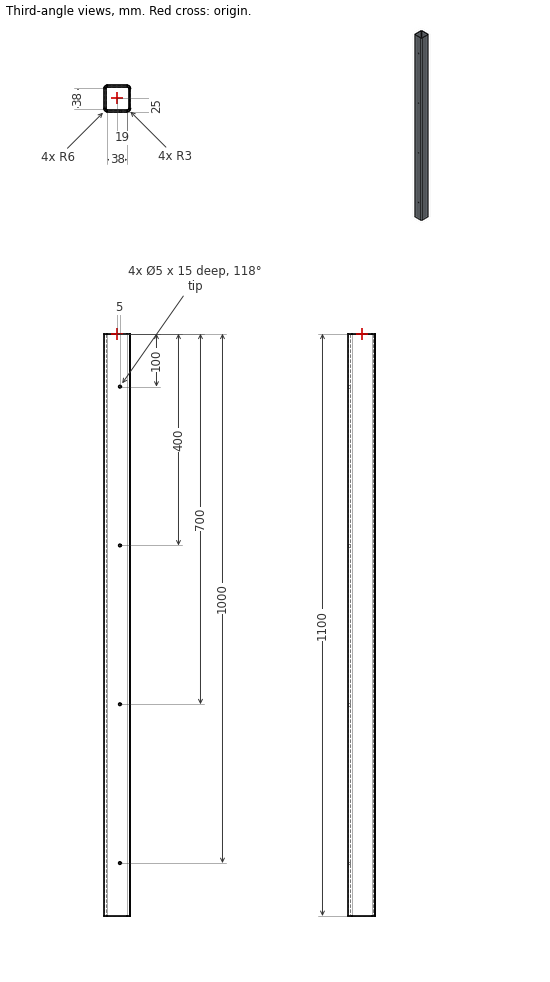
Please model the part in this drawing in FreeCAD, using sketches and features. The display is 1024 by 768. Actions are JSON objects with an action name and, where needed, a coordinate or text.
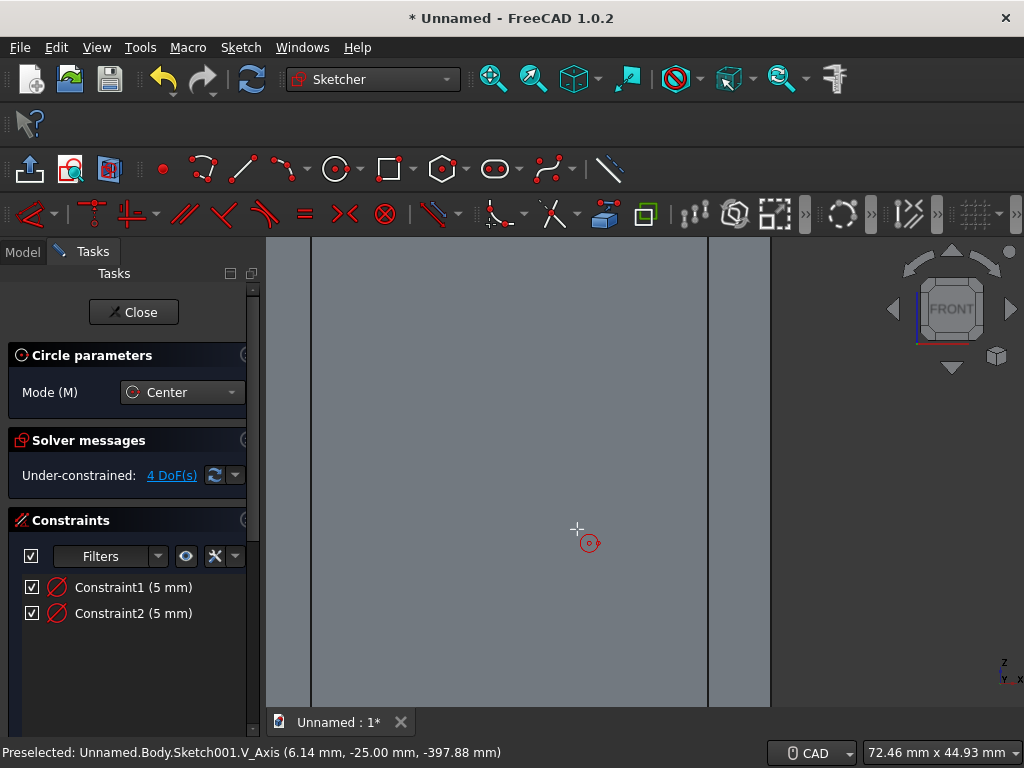
{"action": "scroll", "coordinate": [577, 542], "scroll_direction": "down", "scroll_amount": 17}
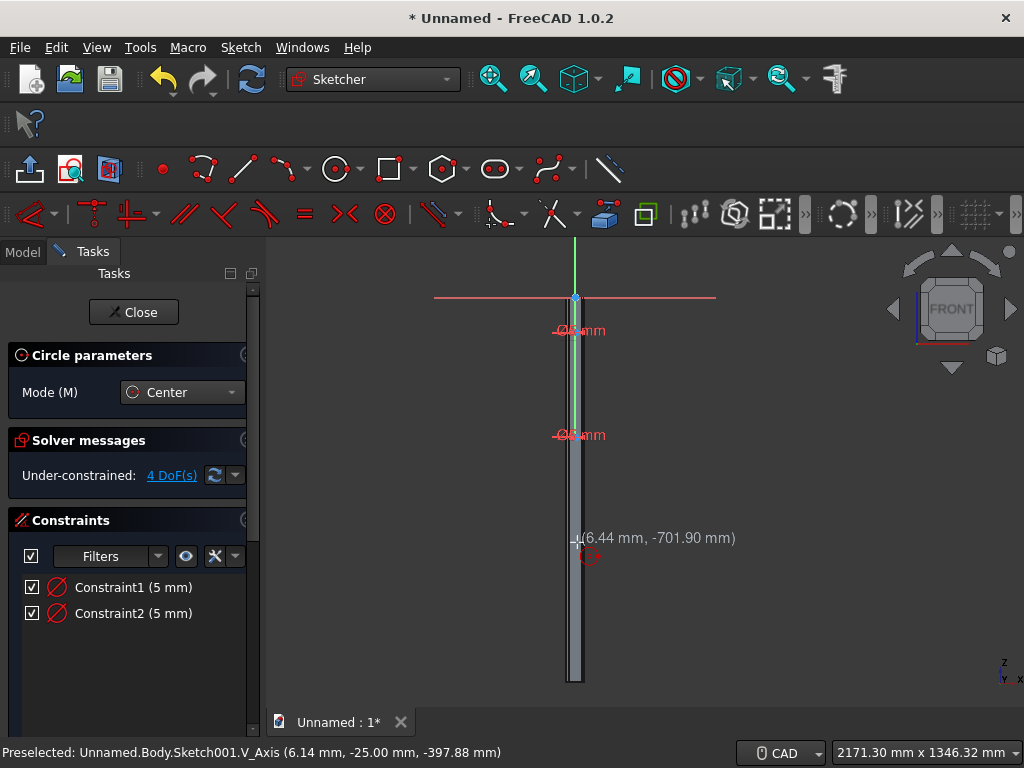
{"action": "scroll", "coordinate": [577, 542], "scroll_direction": "up", "scroll_amount": 12}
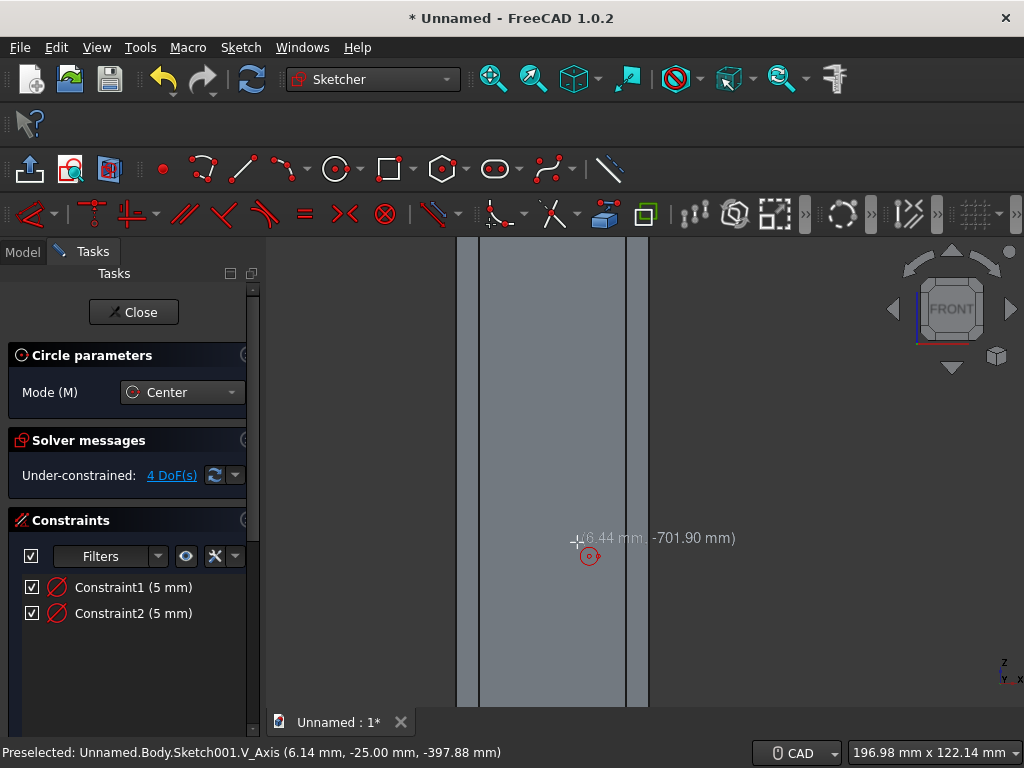
{"action": "left_click", "coordinate": [572, 535]}
{"action": "mouse_move", "coordinate": [579, 529]}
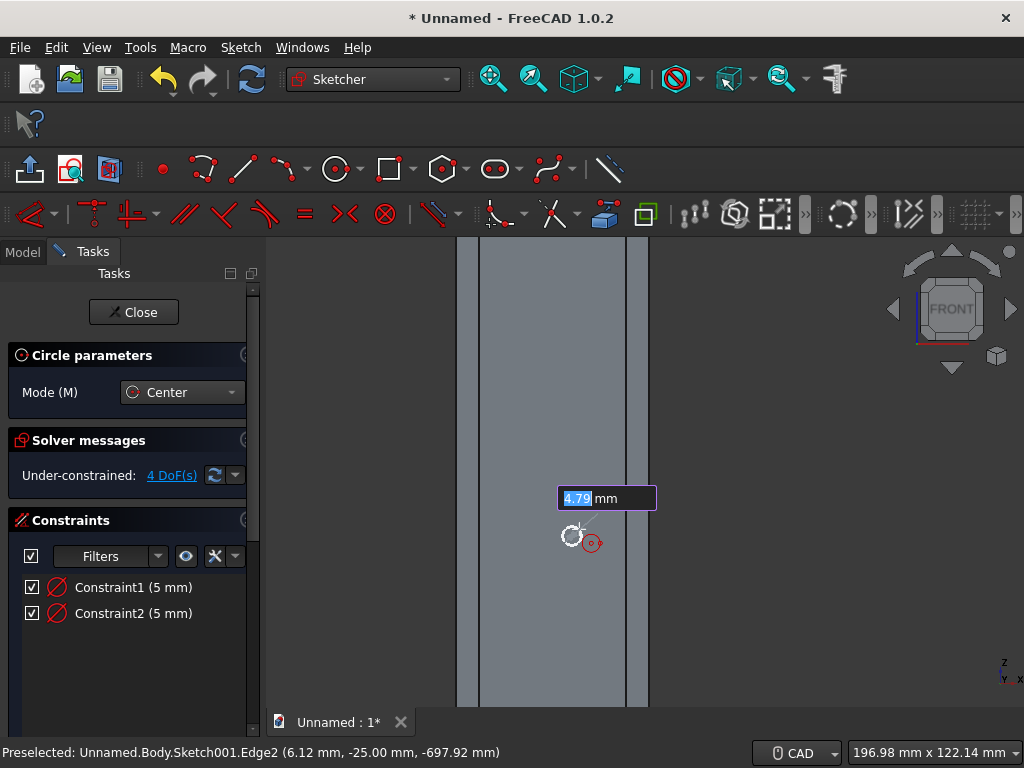
{"action": "type", "text": "5"}
{"action": "key", "text": "Return"}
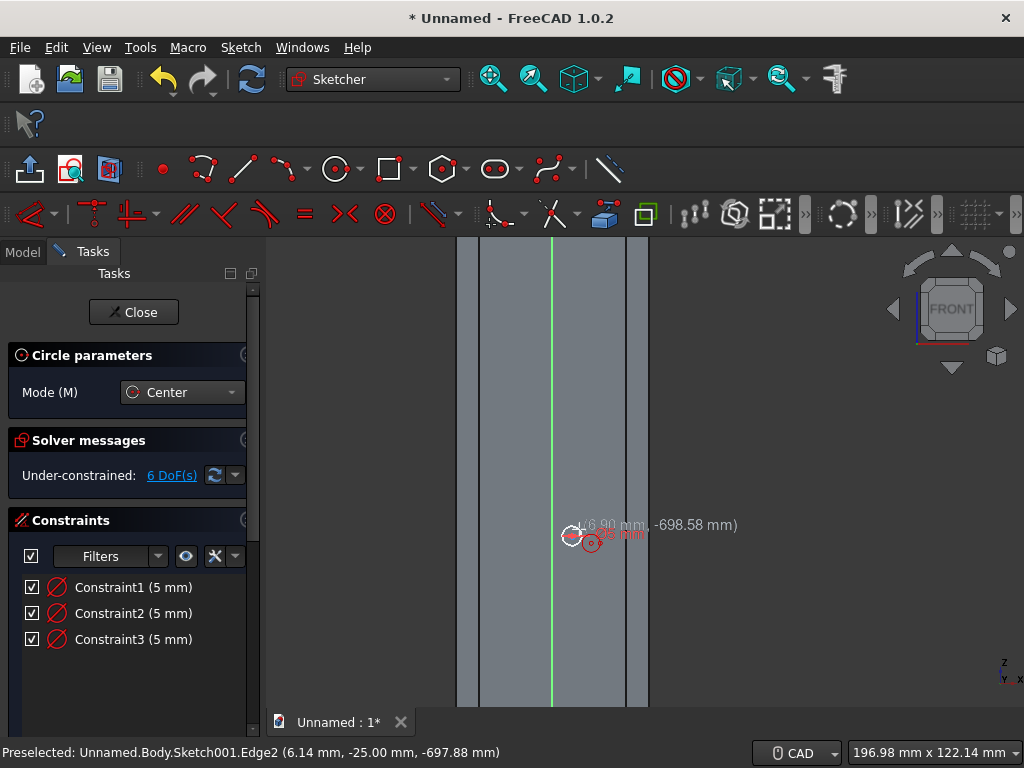
{"action": "scroll", "coordinate": [577, 528], "scroll_direction": "down", "scroll_amount": 13}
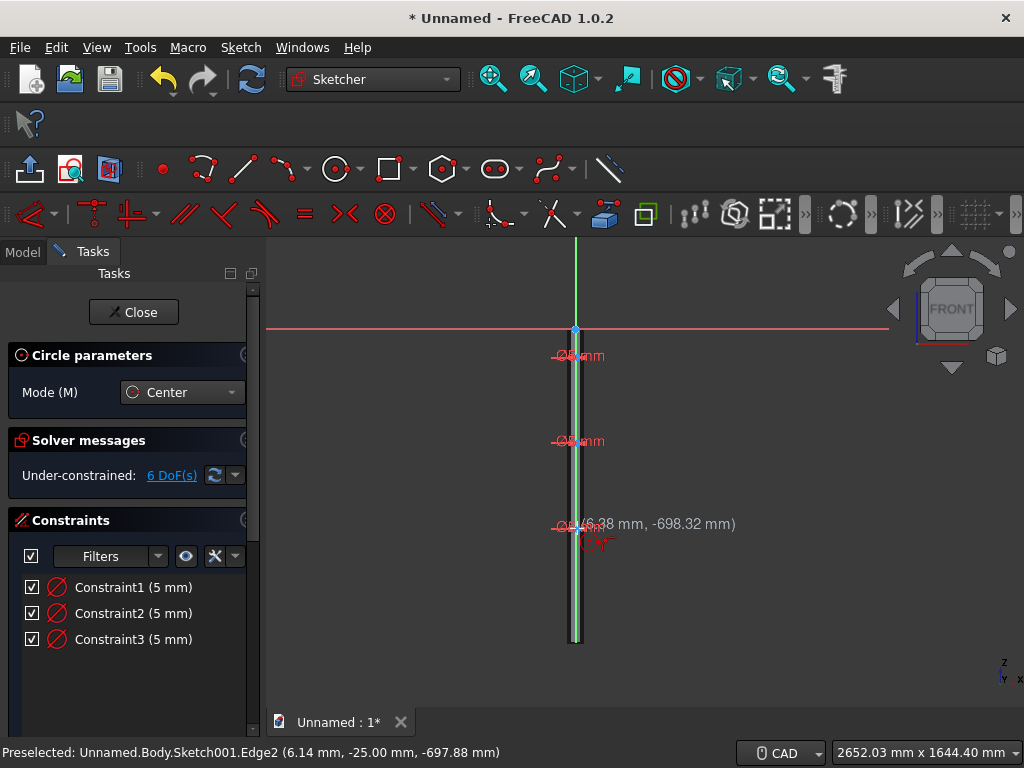
{"action": "scroll", "coordinate": [577, 615], "scroll_direction": "up", "scroll_amount": 18}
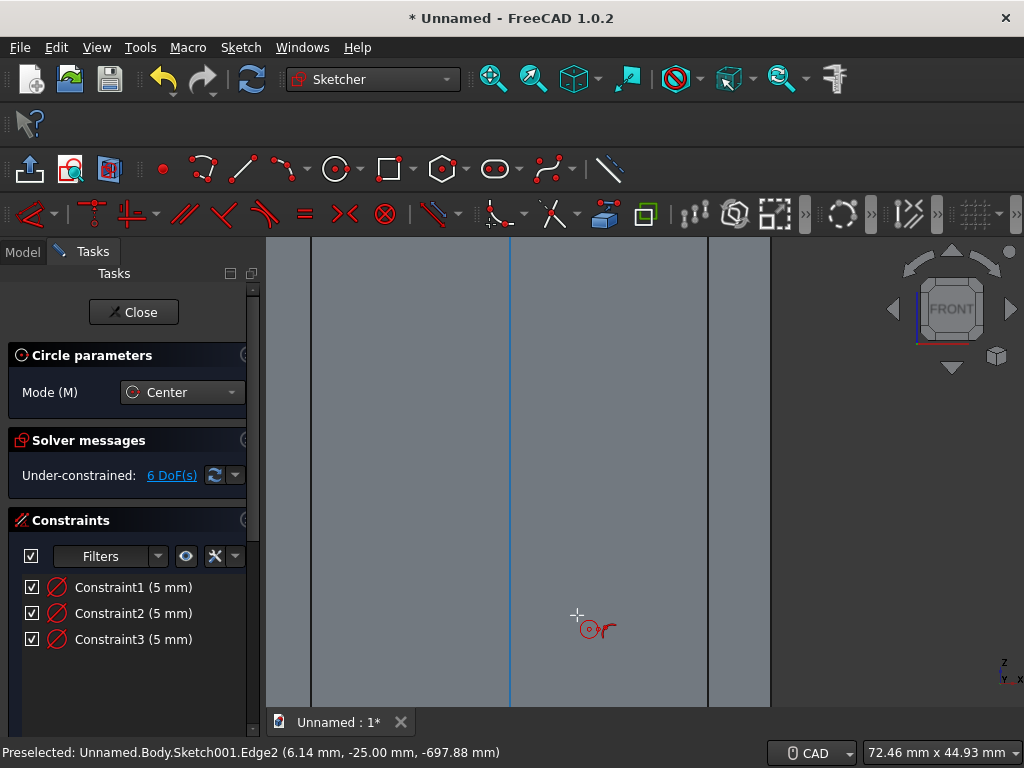
{"action": "scroll", "coordinate": [577, 648], "scroll_direction": "down", "scroll_amount": 17}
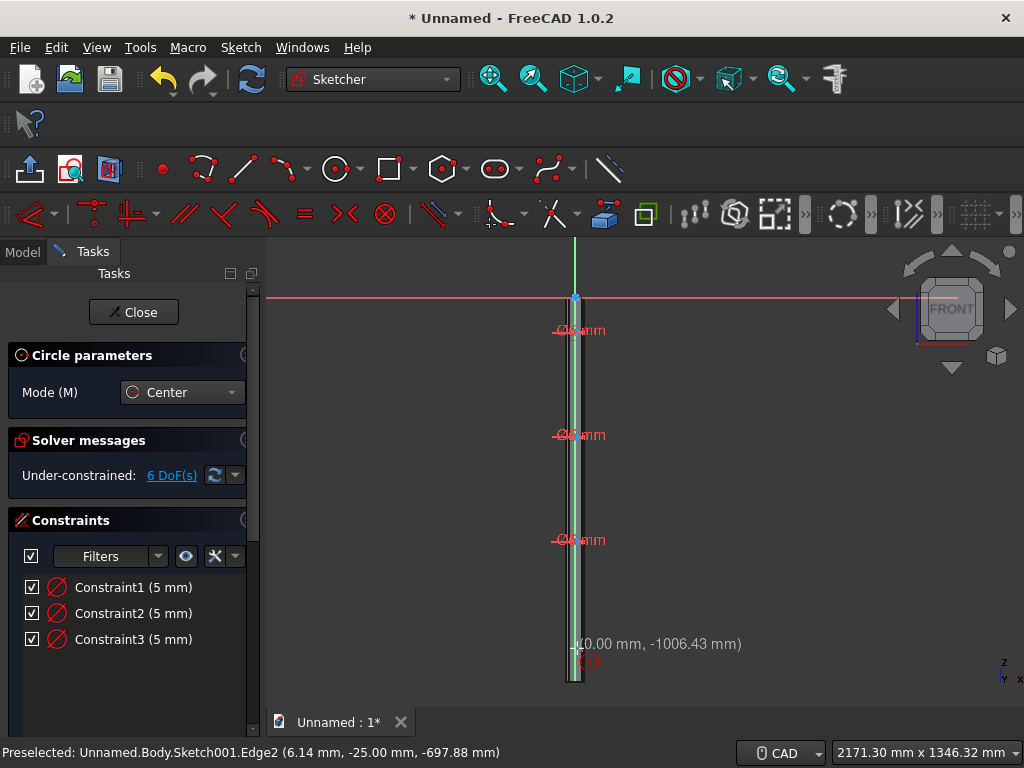
{"action": "scroll", "coordinate": [577, 647], "scroll_direction": "up", "scroll_amount": 12}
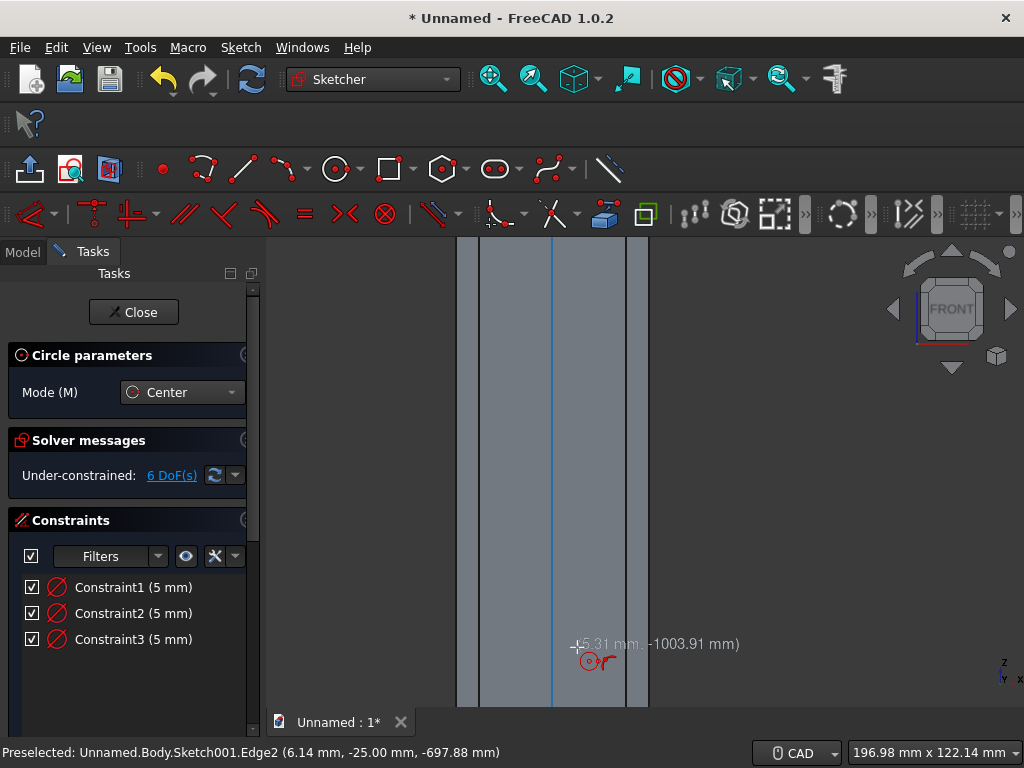
{"action": "left_click", "coordinate": [572, 634]}
{"action": "mouse_move", "coordinate": [579, 627]}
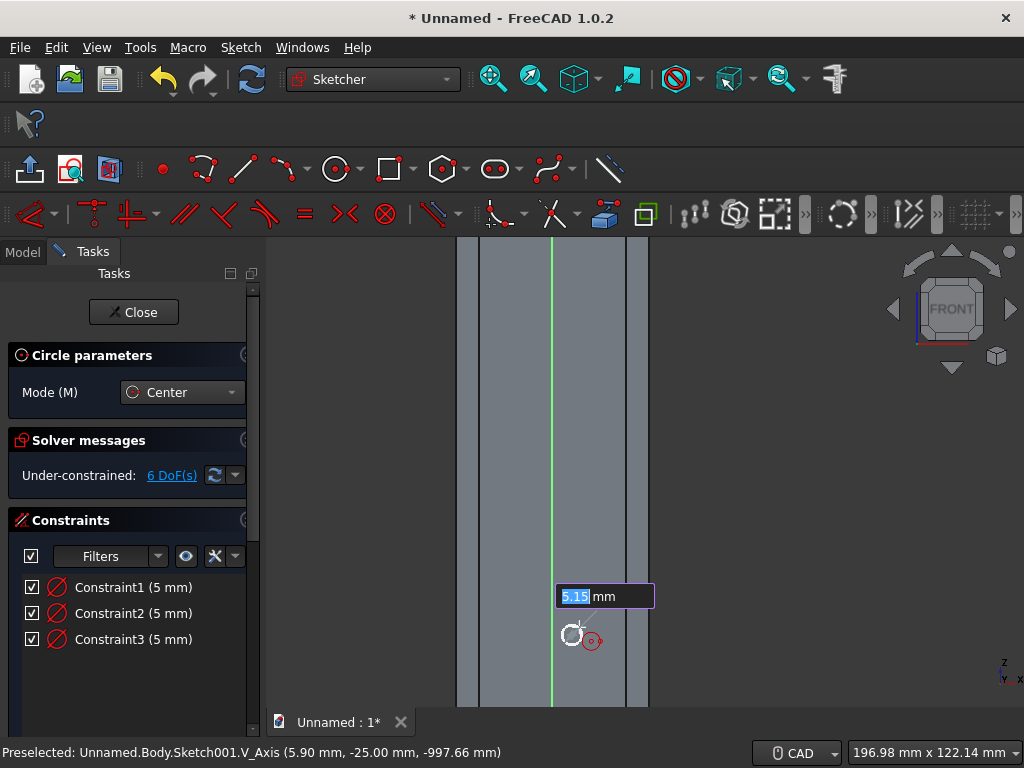
{"action": "type", "text": "5"}
{"action": "key", "text": "Return"}
{"action": "key", "text": "Escape"}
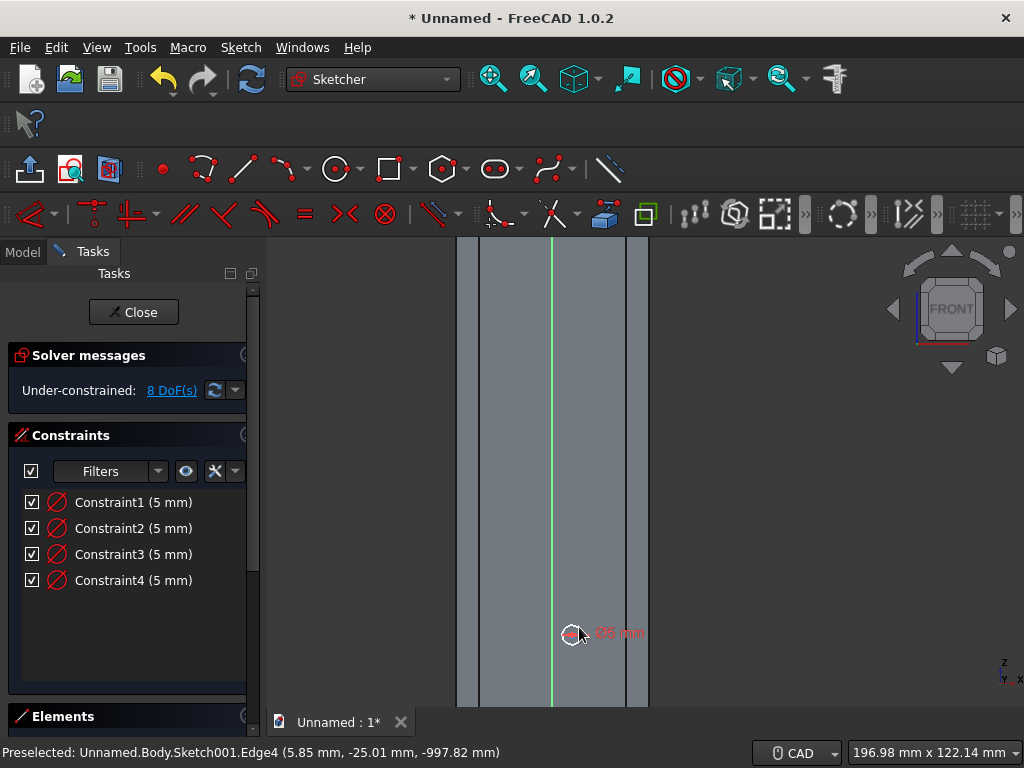
{"action": "scroll", "coordinate": [577, 613], "scroll_direction": "down", "scroll_amount": 13}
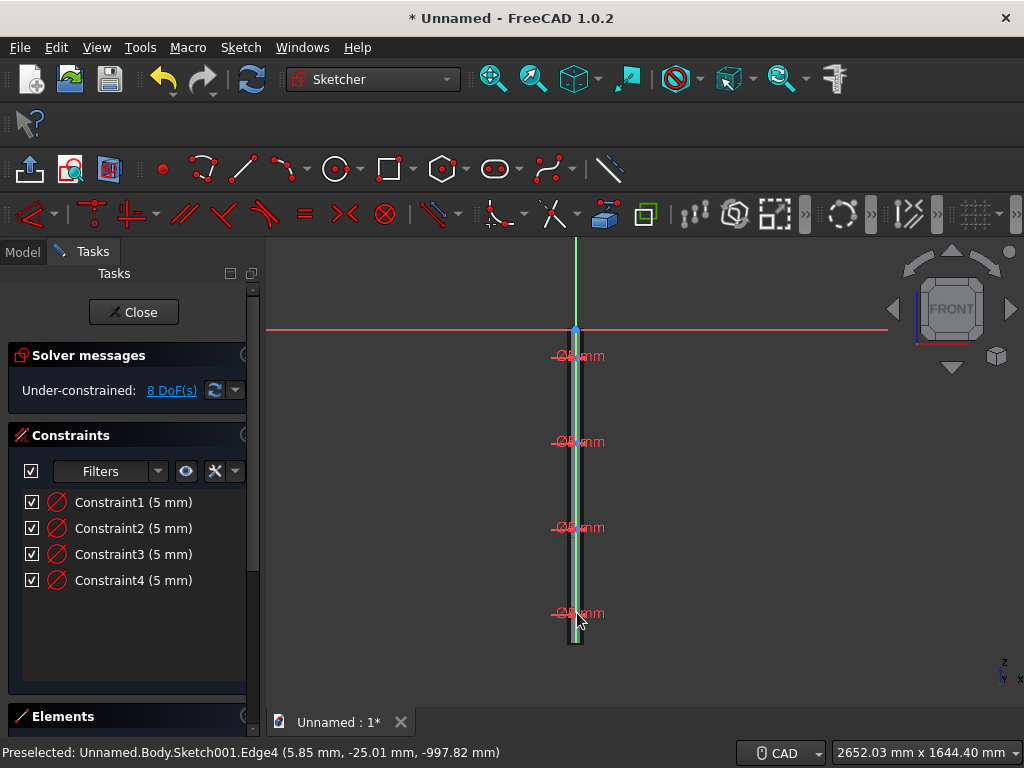
{"action": "scroll", "coordinate": [577, 358], "scroll_direction": "up", "scroll_amount": 17}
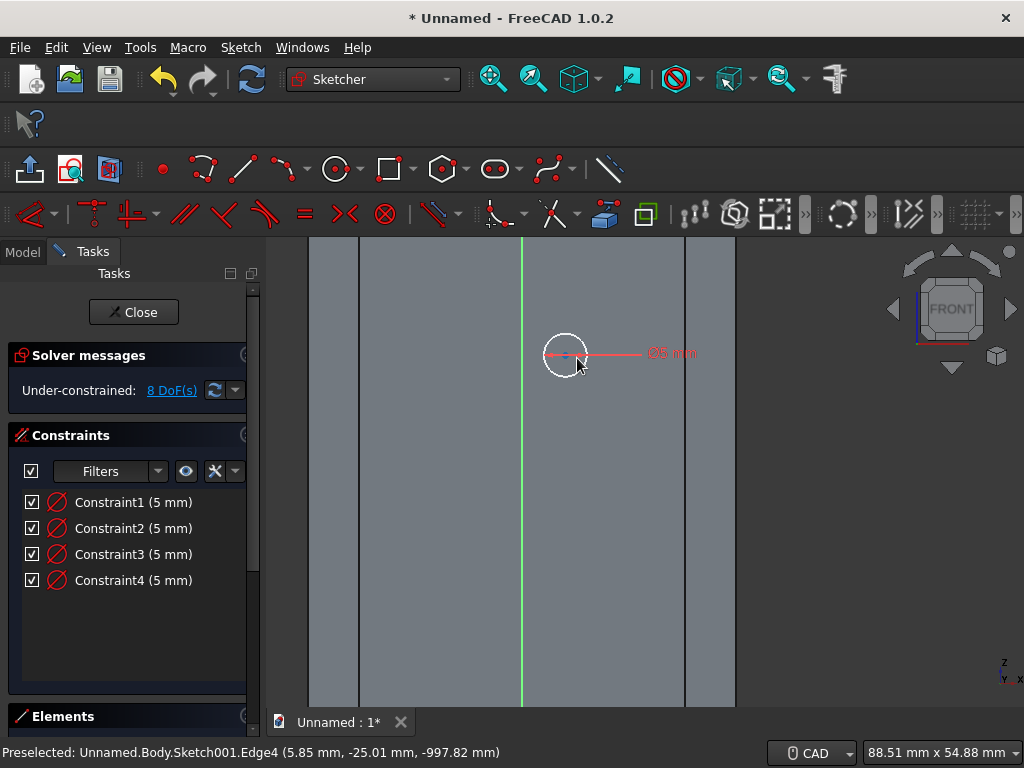
{"action": "left_click", "coordinate": [565, 355]}